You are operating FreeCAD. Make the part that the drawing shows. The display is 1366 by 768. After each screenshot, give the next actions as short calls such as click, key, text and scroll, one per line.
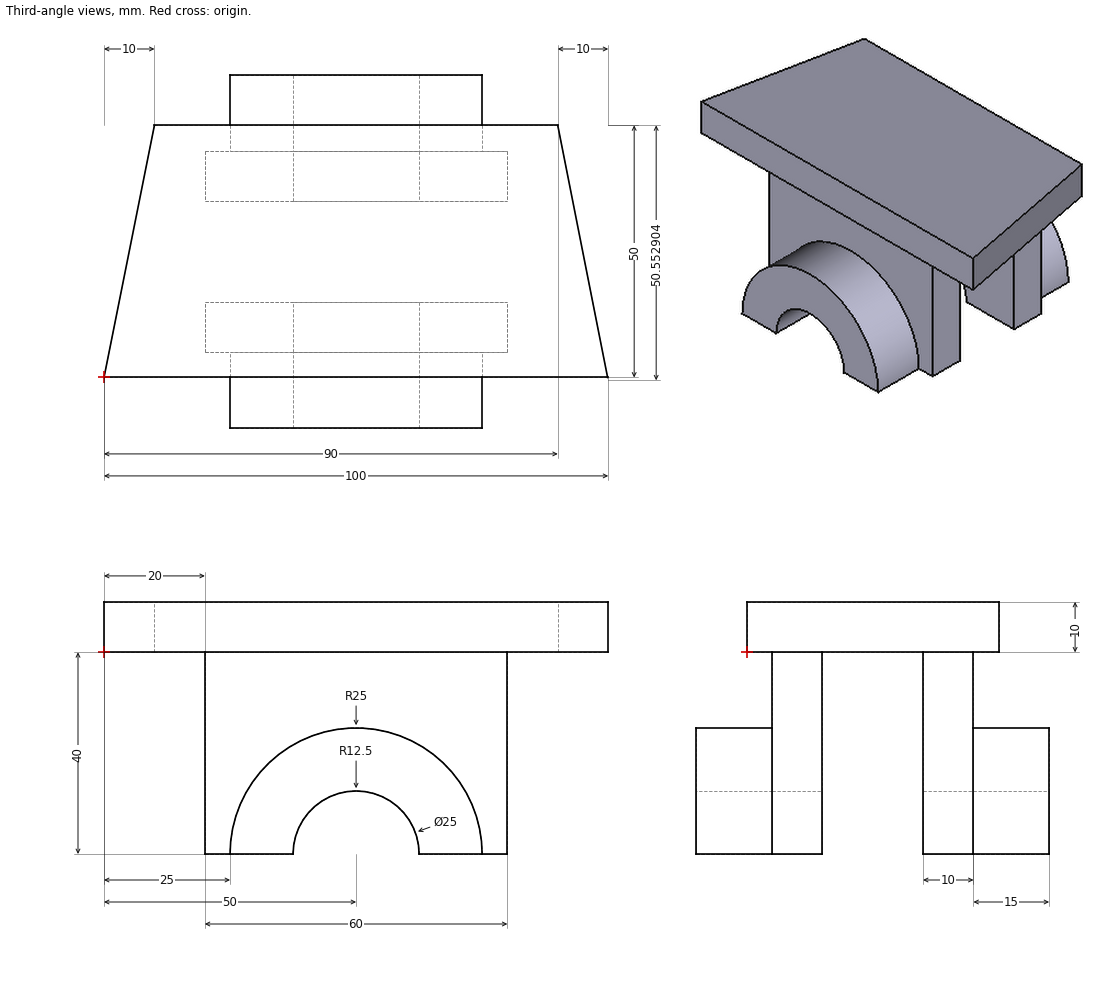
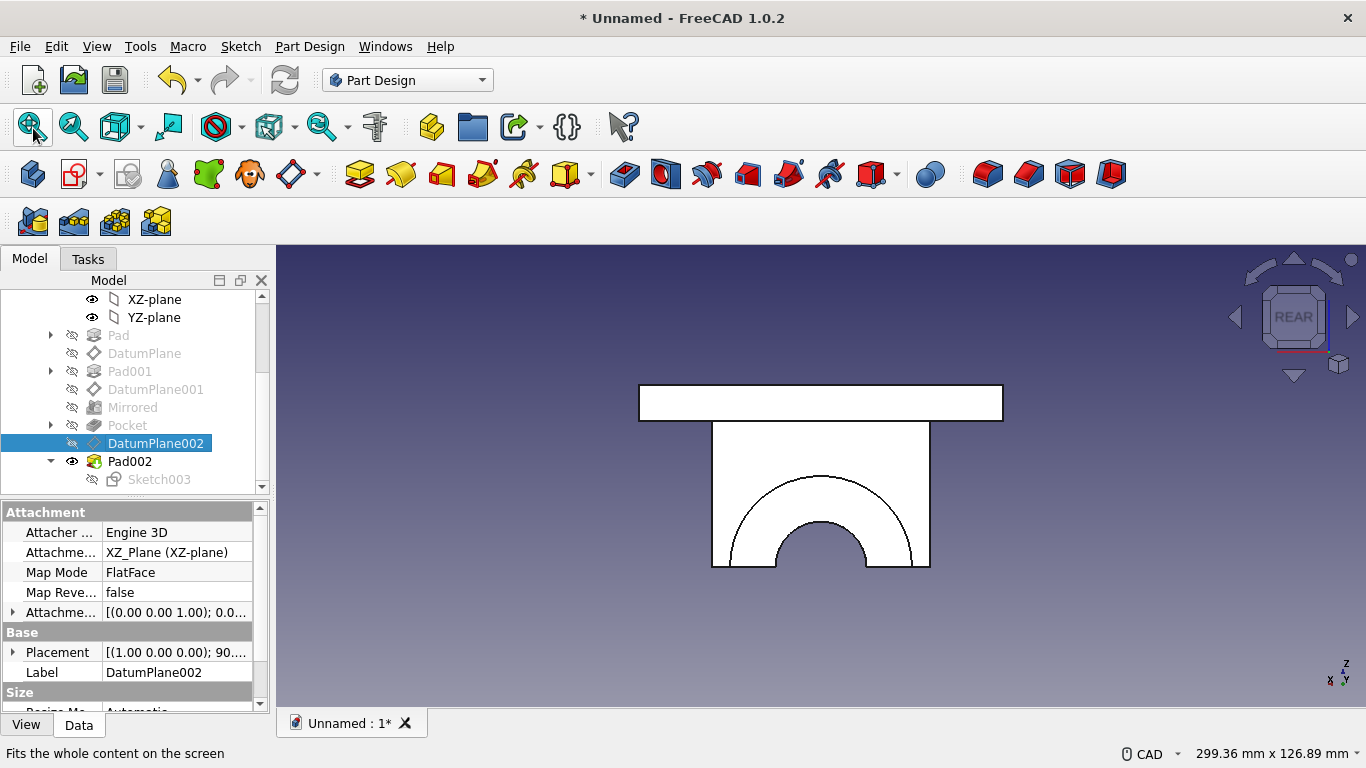
scroll(161, 385, down, 3)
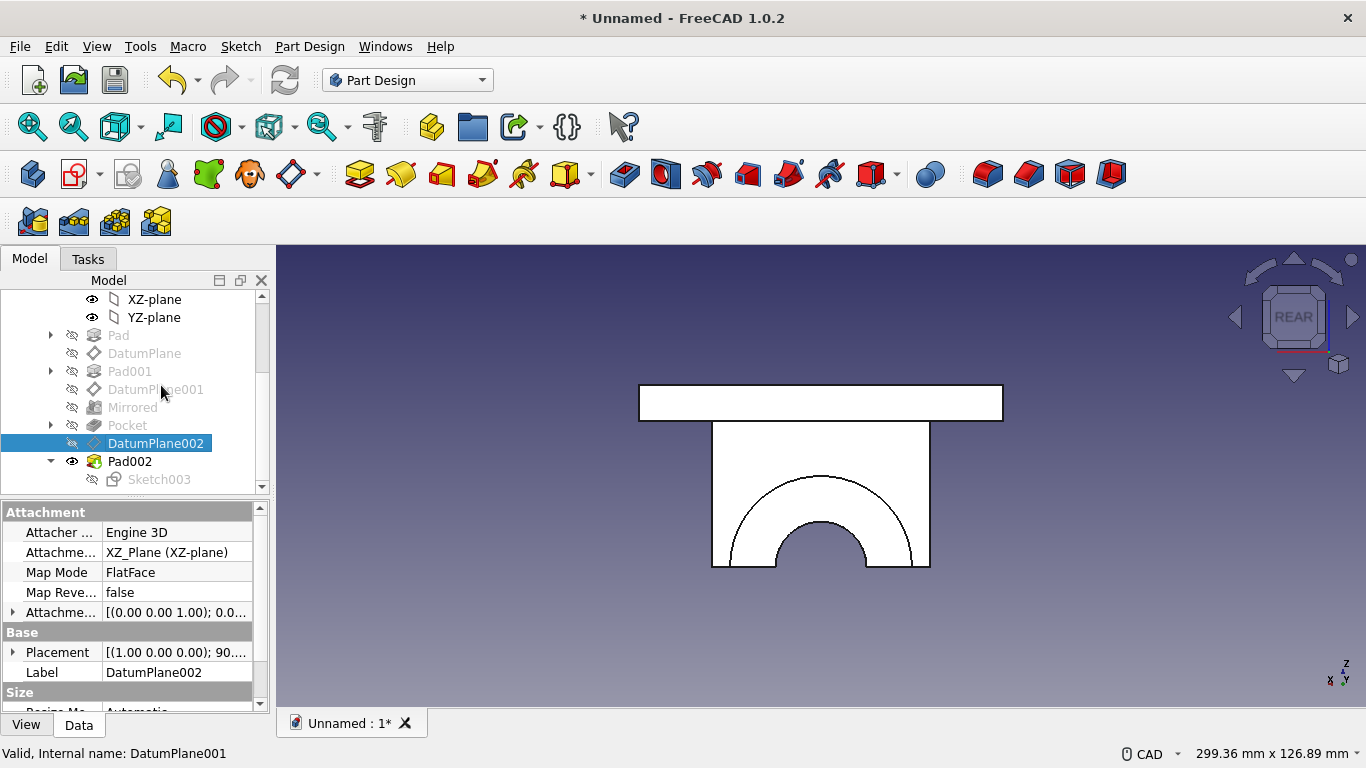
scroll(161, 385, up, 15)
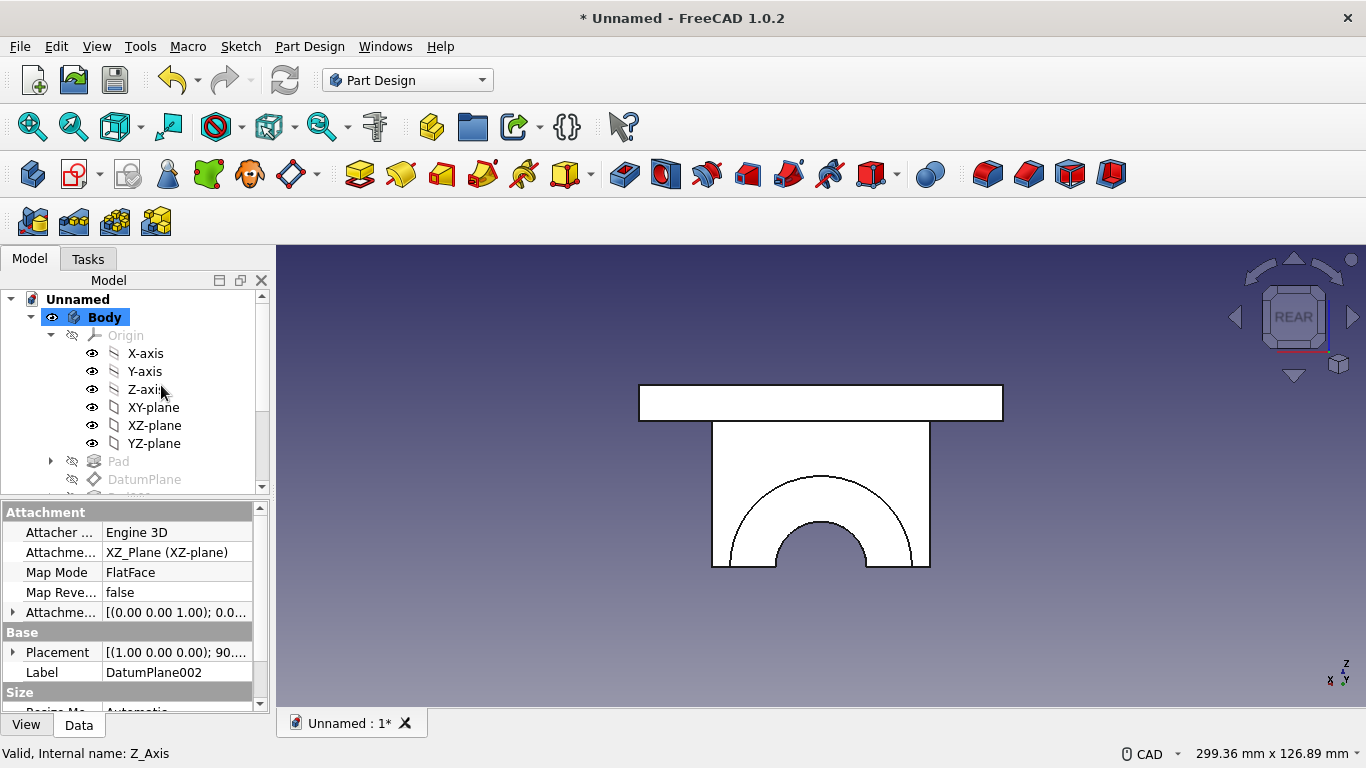
click(137, 425)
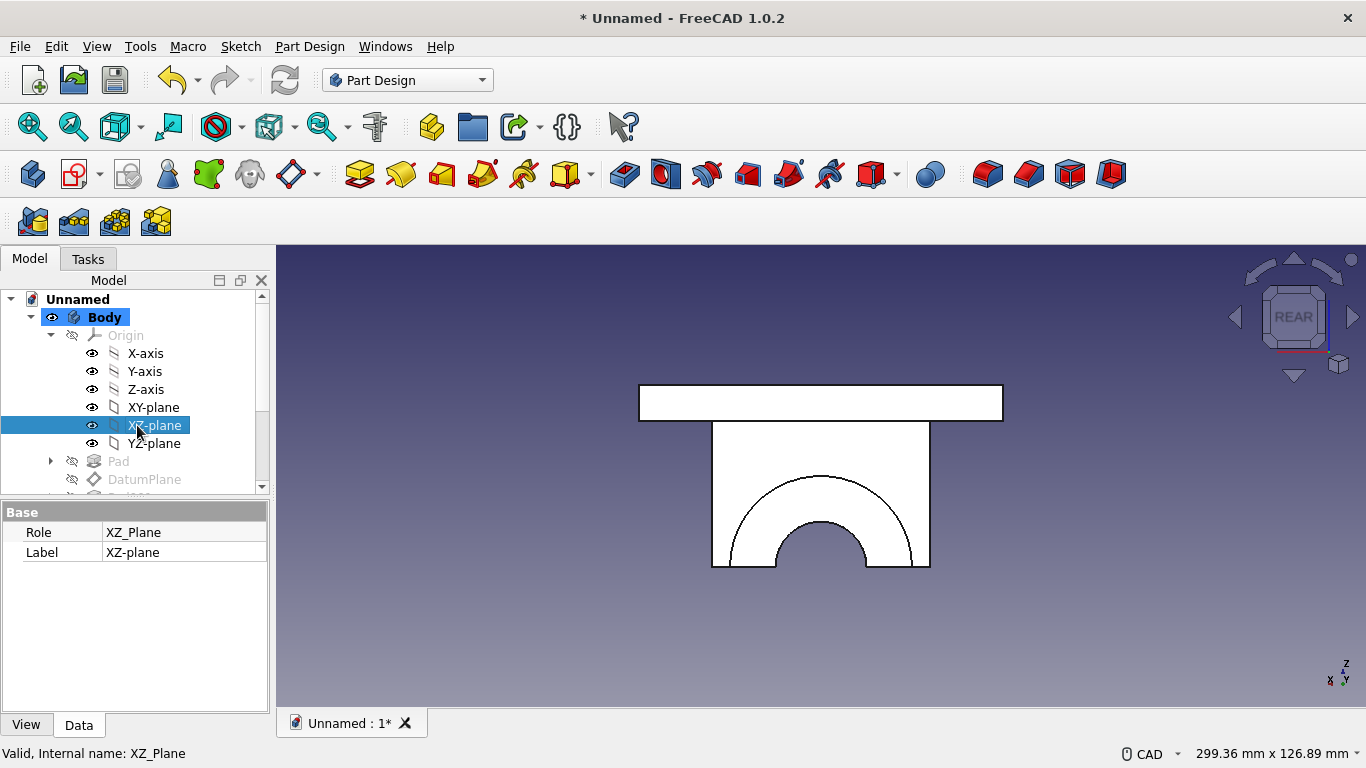
click(290, 174)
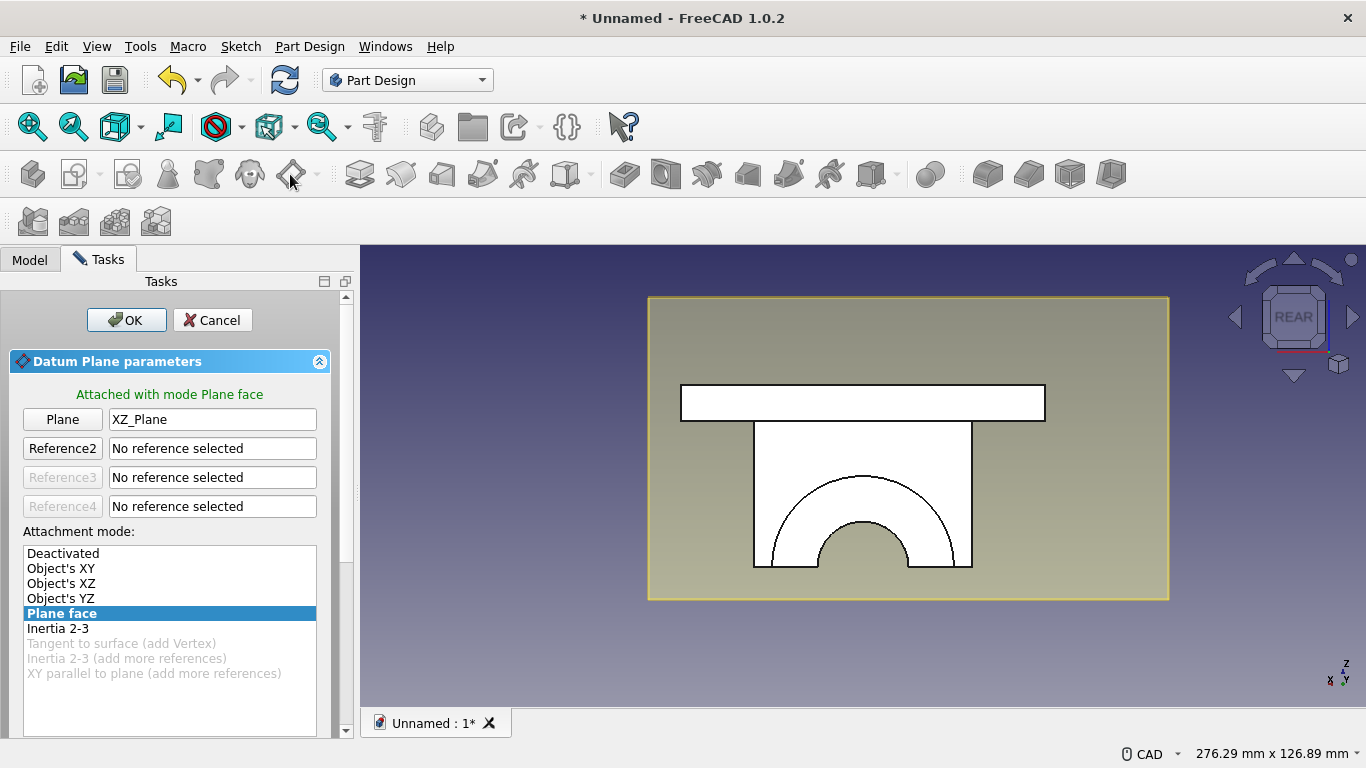
scroll(346, 514, down, 4)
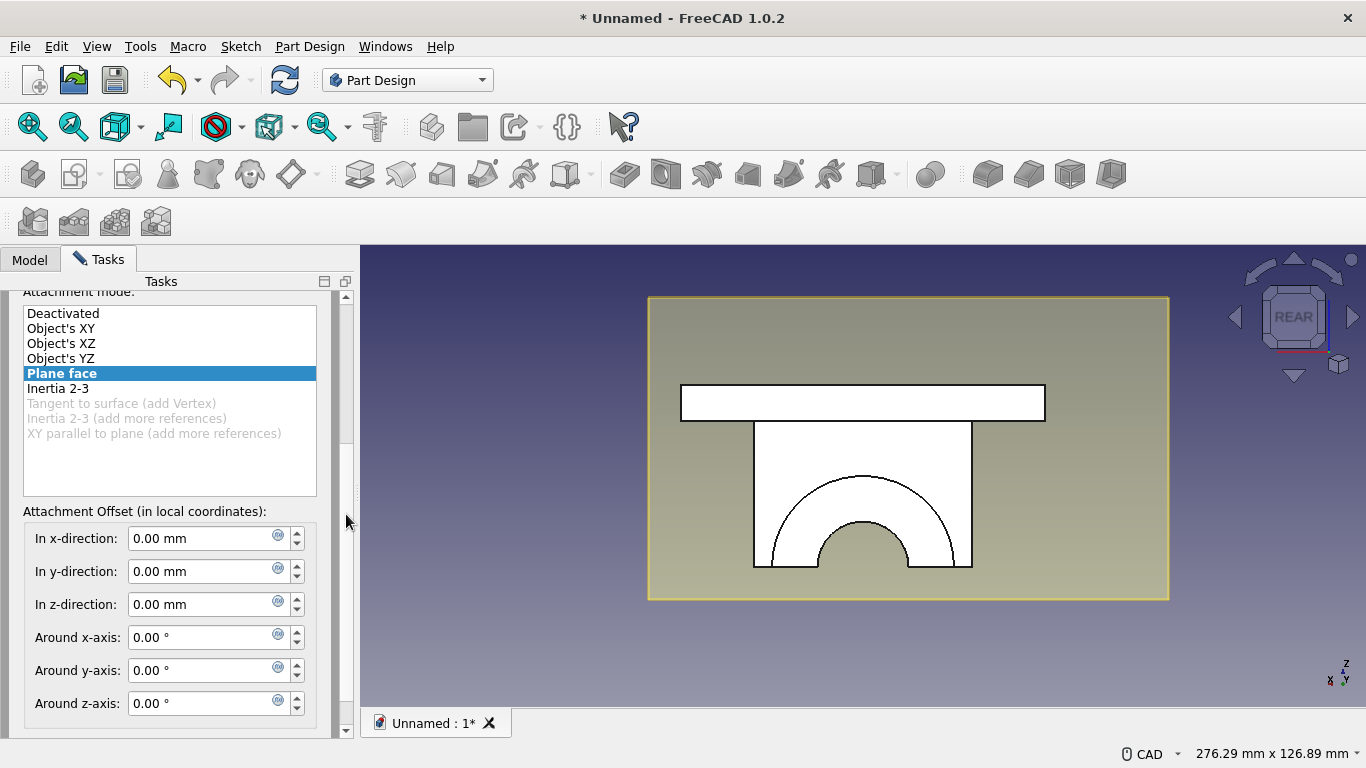
triple_click(210, 604)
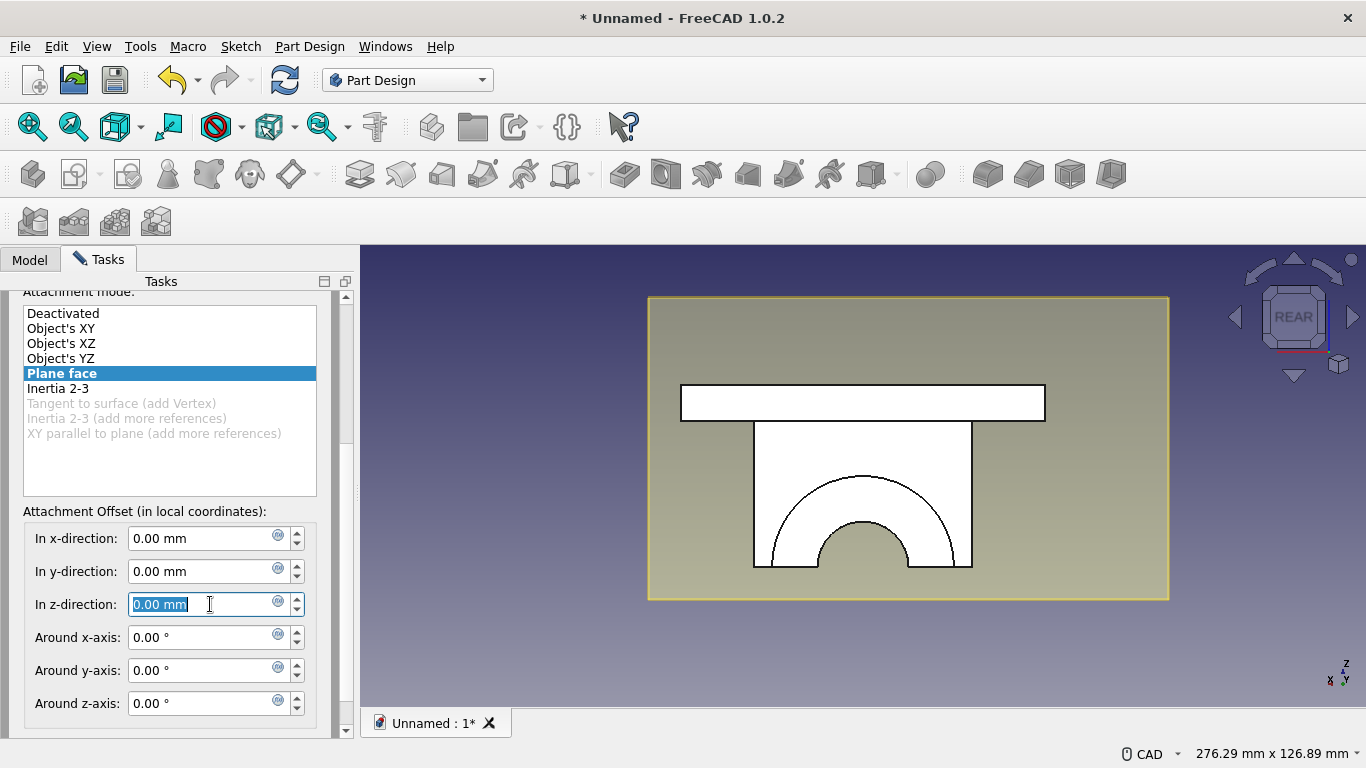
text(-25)
key(Tab)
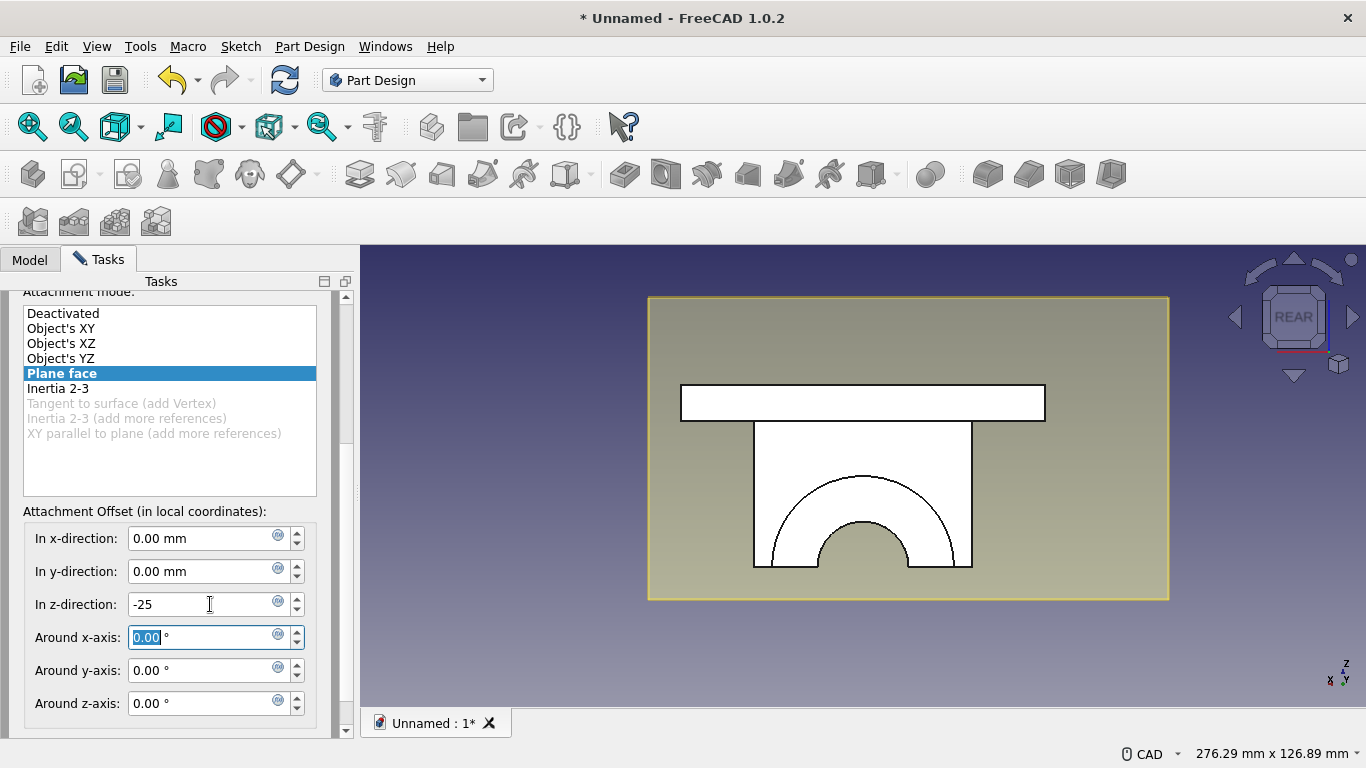
scroll(346, 514, up, 5)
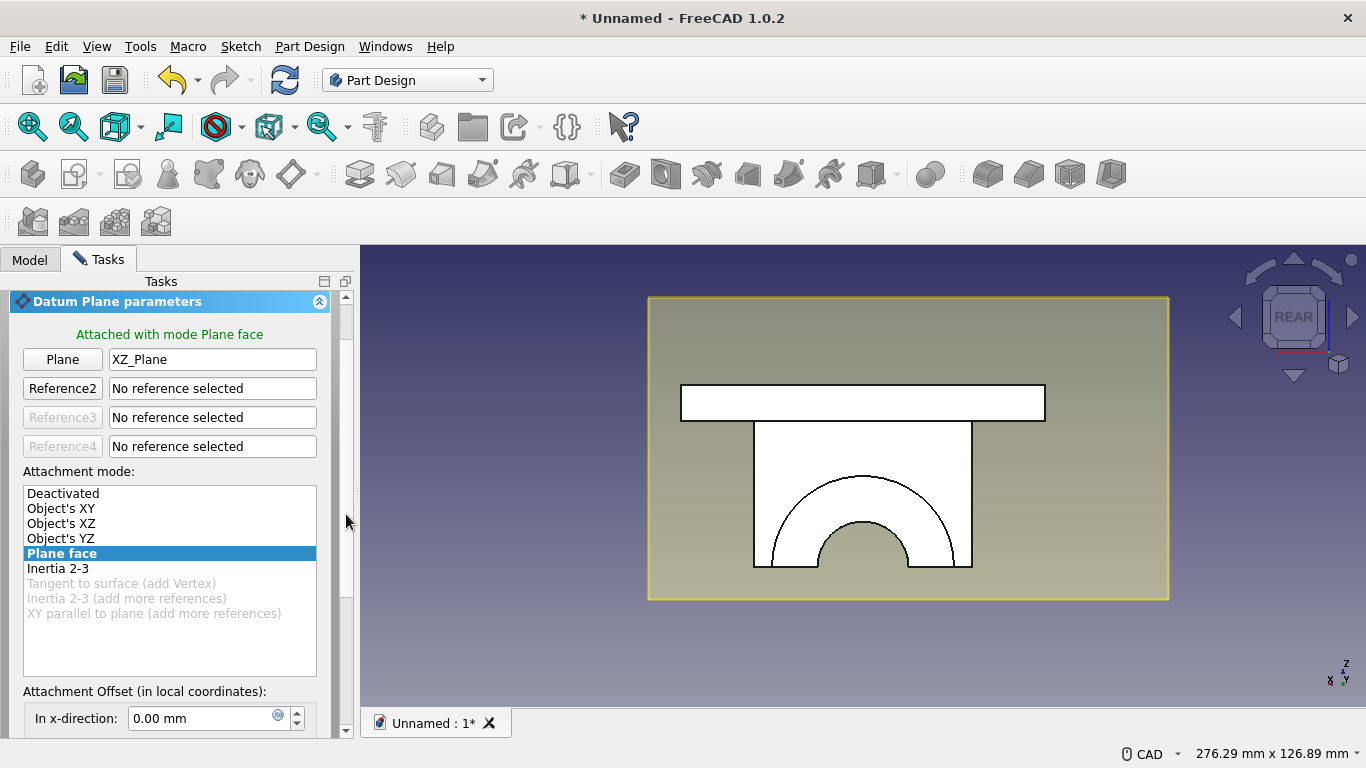
click(127, 320)